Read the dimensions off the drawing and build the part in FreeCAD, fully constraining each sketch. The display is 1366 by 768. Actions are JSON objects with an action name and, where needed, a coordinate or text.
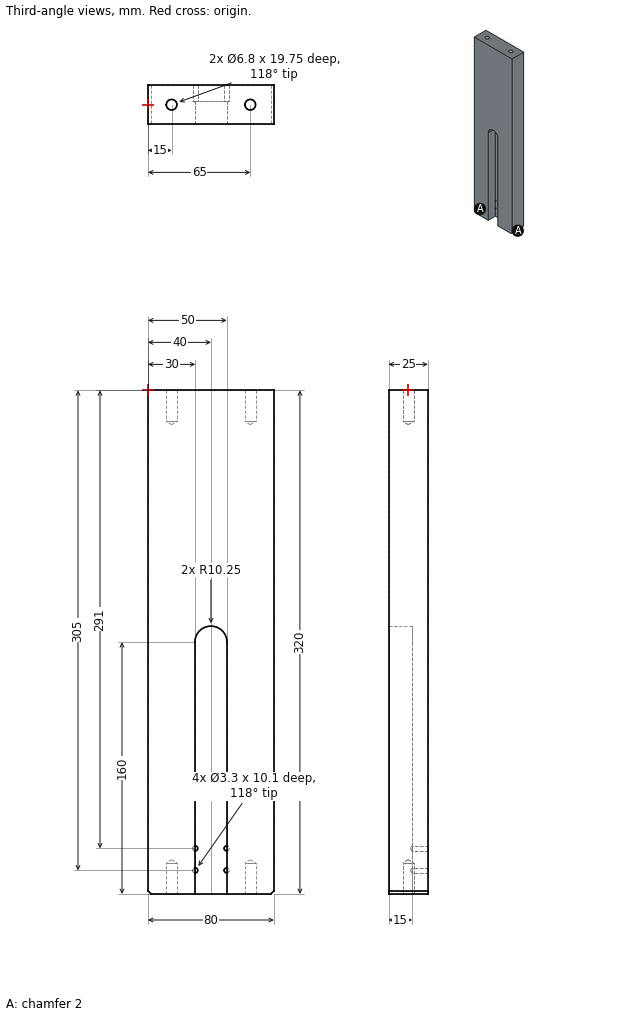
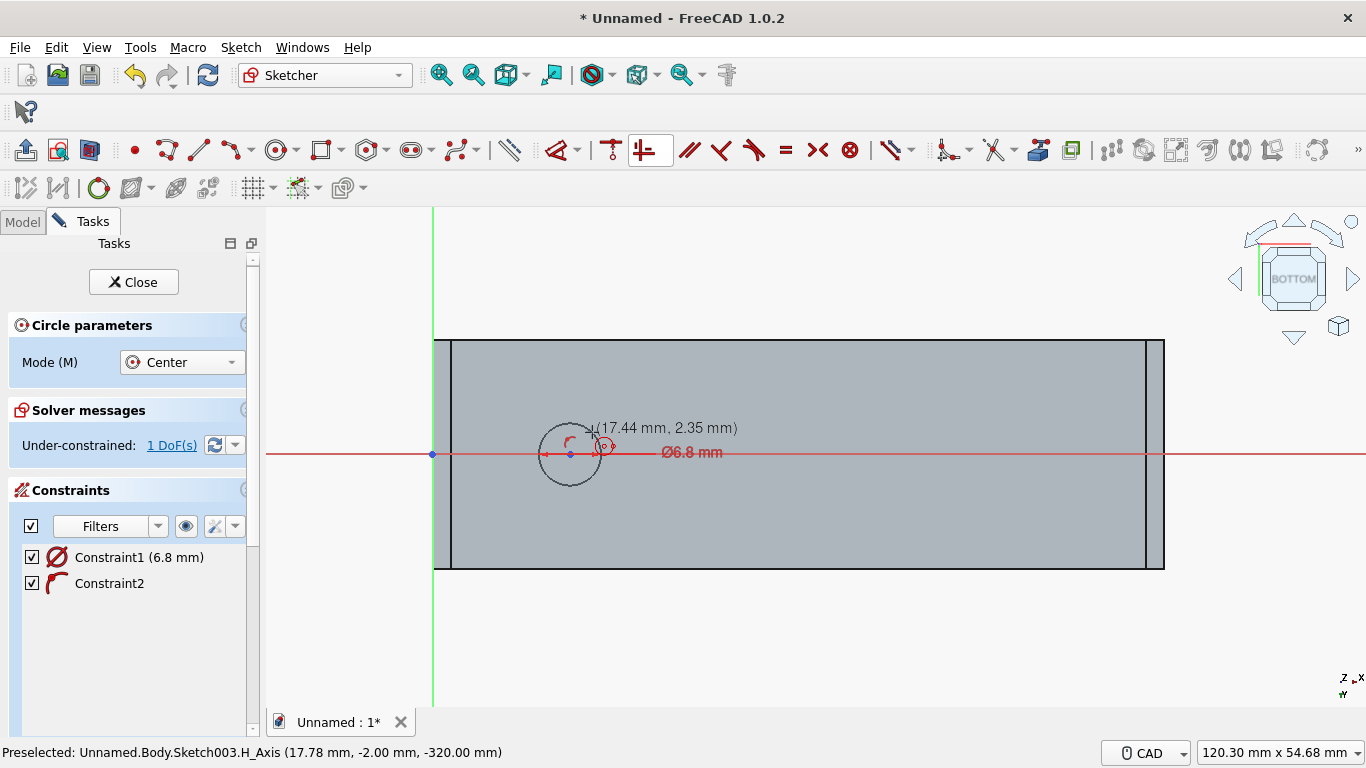
{"action": "left_click", "coordinate": [1027, 454]}
{"action": "mouse_move", "coordinate": [1049, 432]}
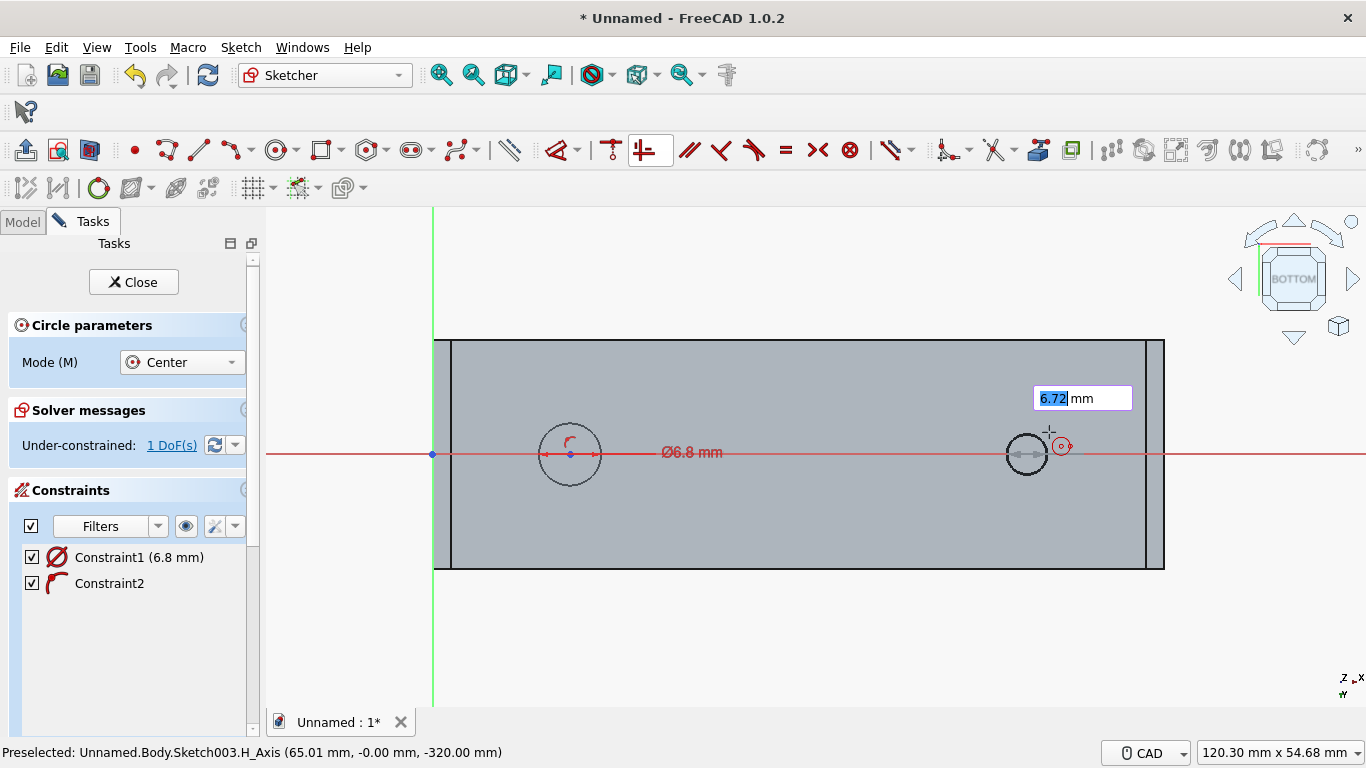
{"action": "type", "text": "6.8"}
{"action": "key", "text": "Return"}
{"action": "key", "text": "Escape"}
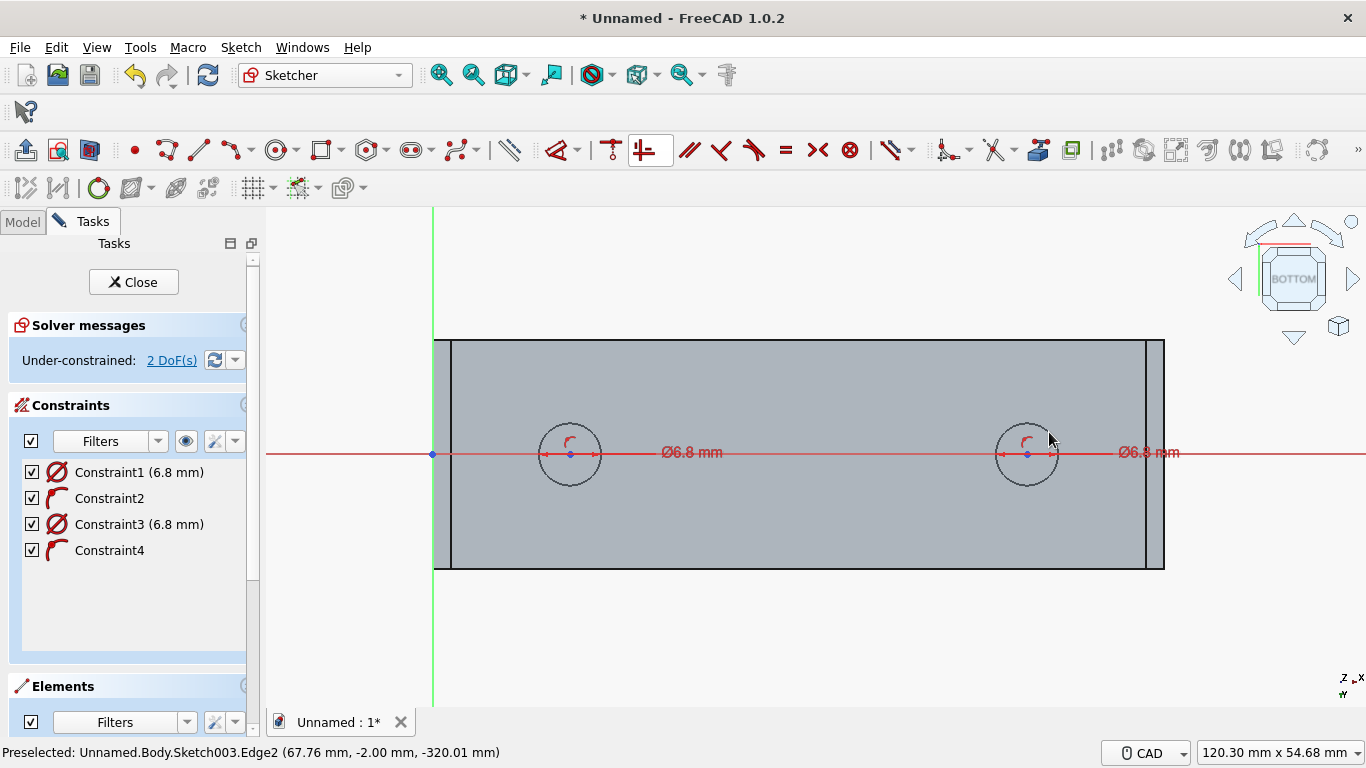
{"action": "key", "text": "d"}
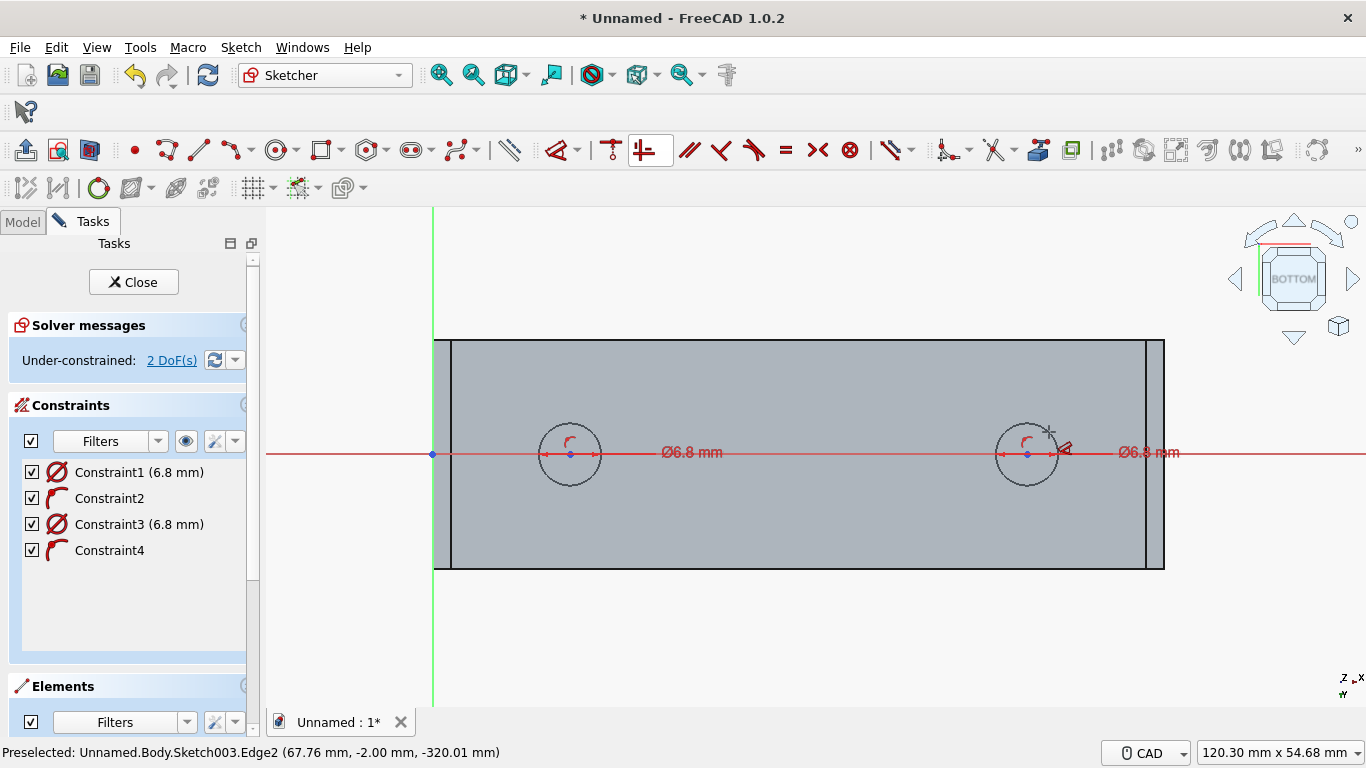
{"action": "left_click", "coordinate": [570, 454]}
{"action": "left_click", "coordinate": [501, 488]}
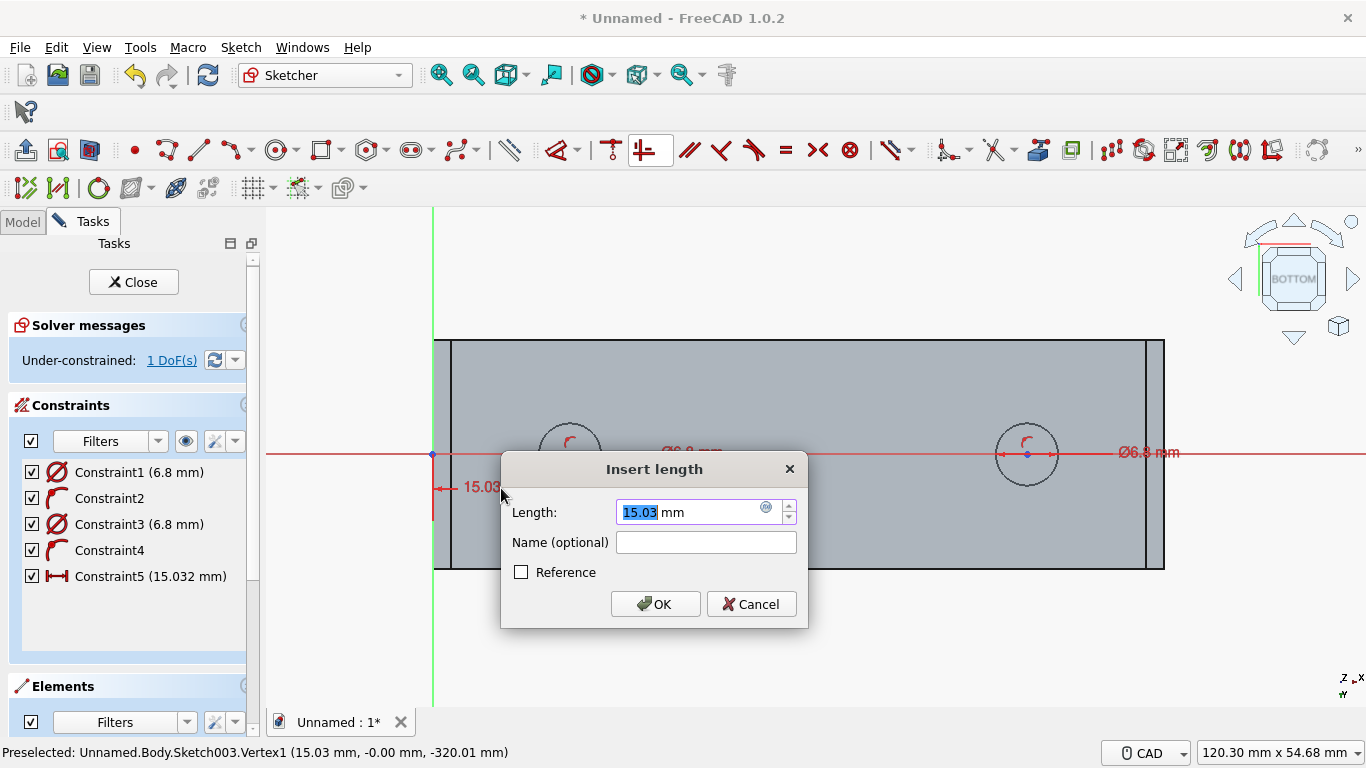
{"action": "type", "text": "15"}
{"action": "key", "text": "Return"}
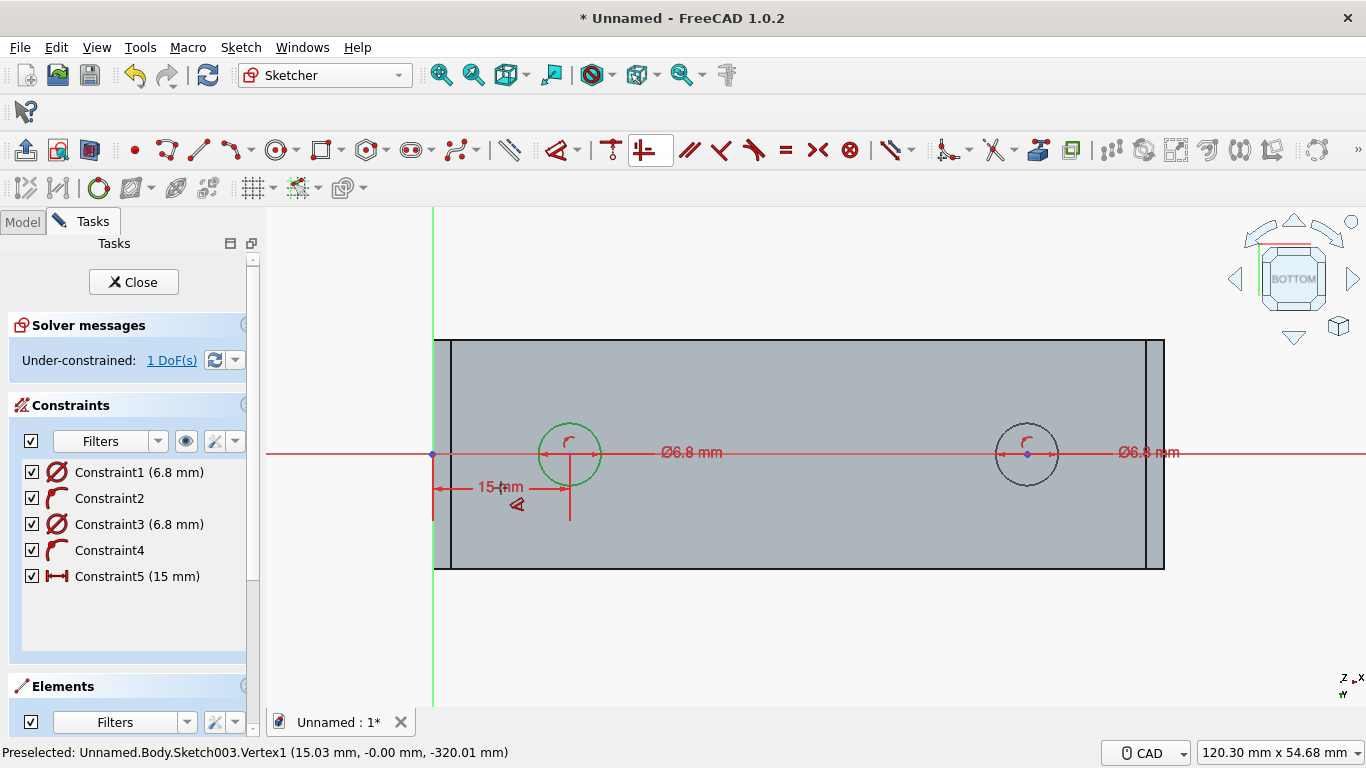
{"action": "left_click", "coordinate": [1027, 454]}
{"action": "left_click", "coordinate": [730, 488]}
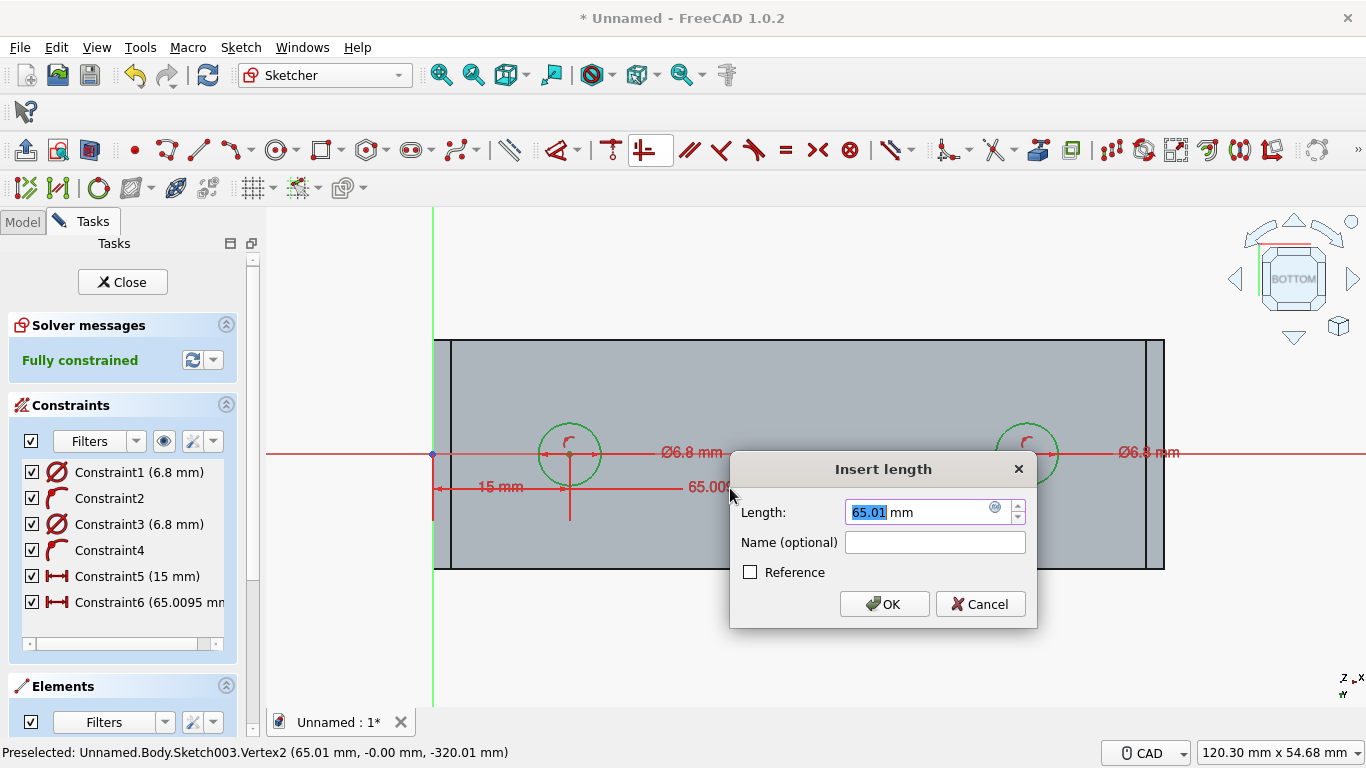
{"action": "type", "text": "65"}
{"action": "key", "text": "Return"}
{"action": "key", "text": "Escape"}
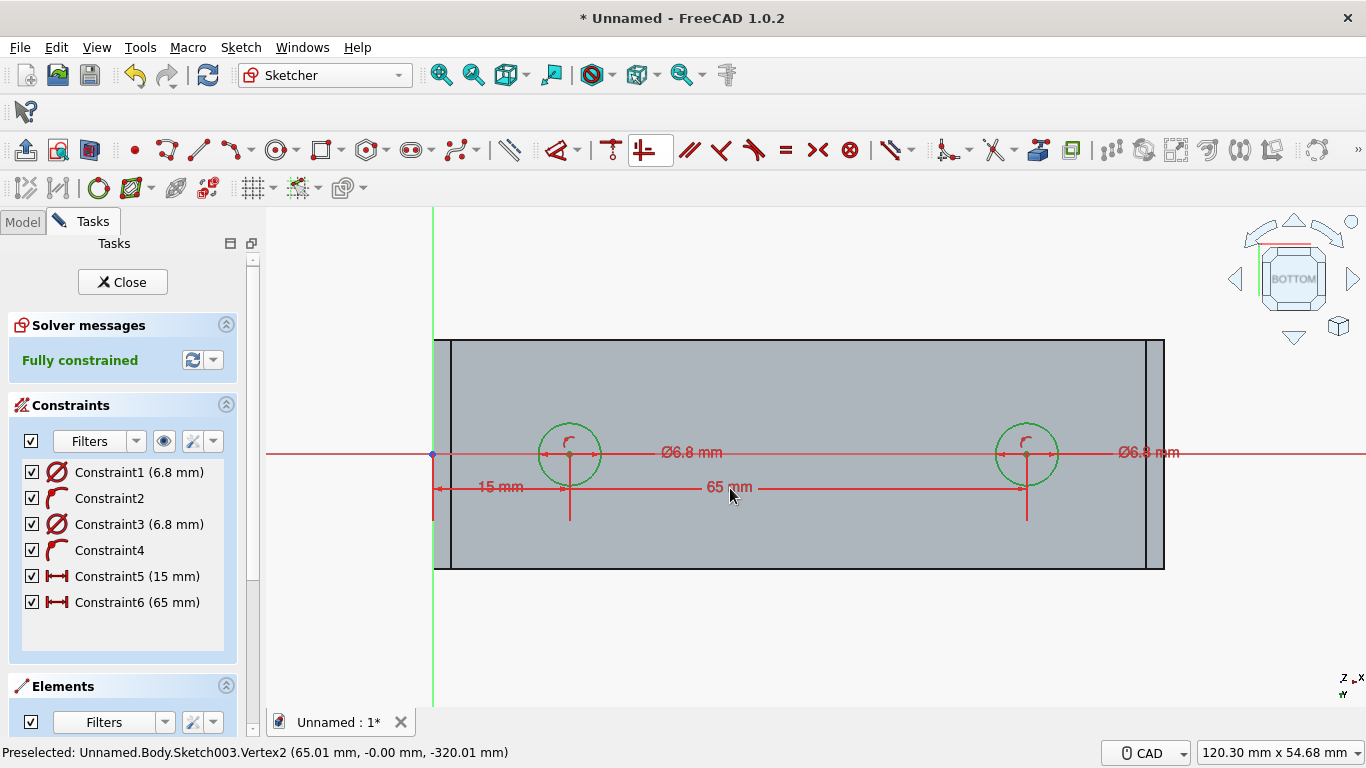
{"action": "left_click", "coordinate": [123, 282]}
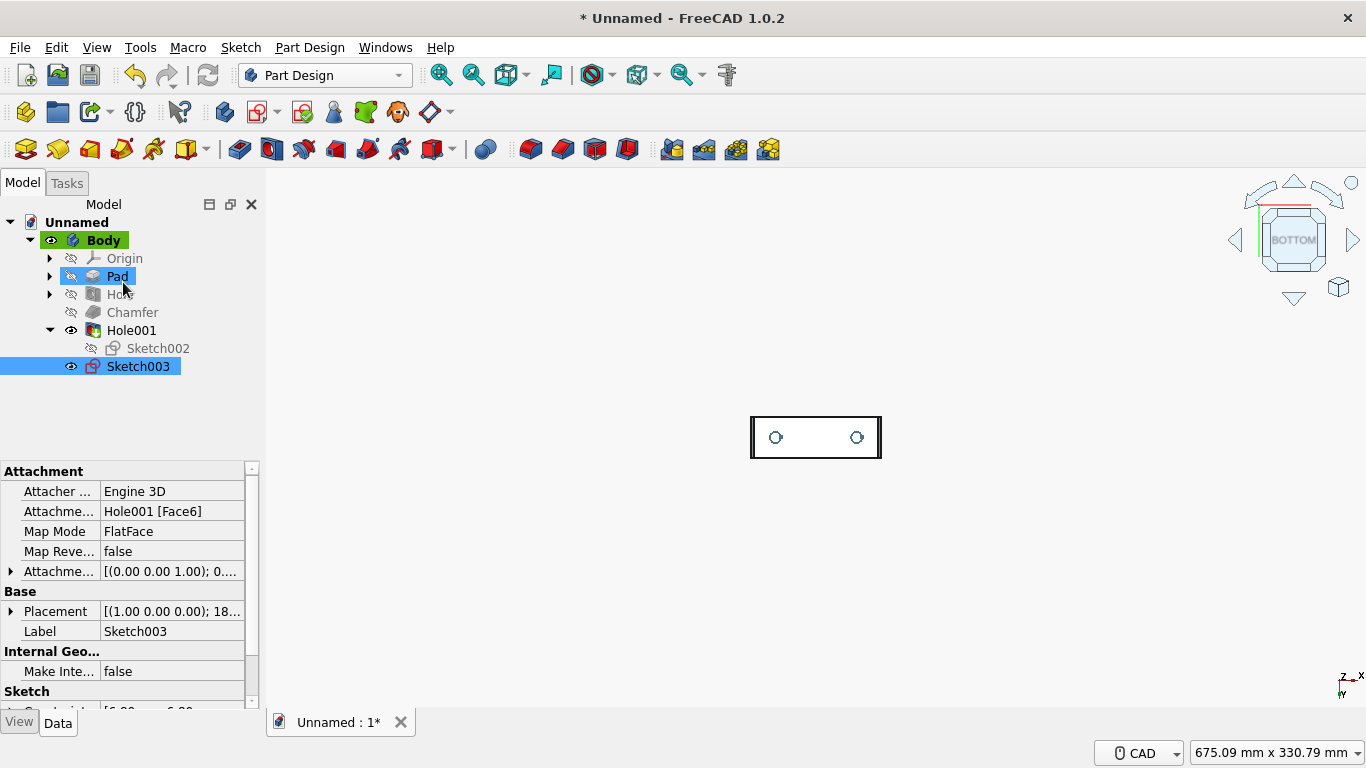
{"action": "left_click", "coordinate": [272, 150]}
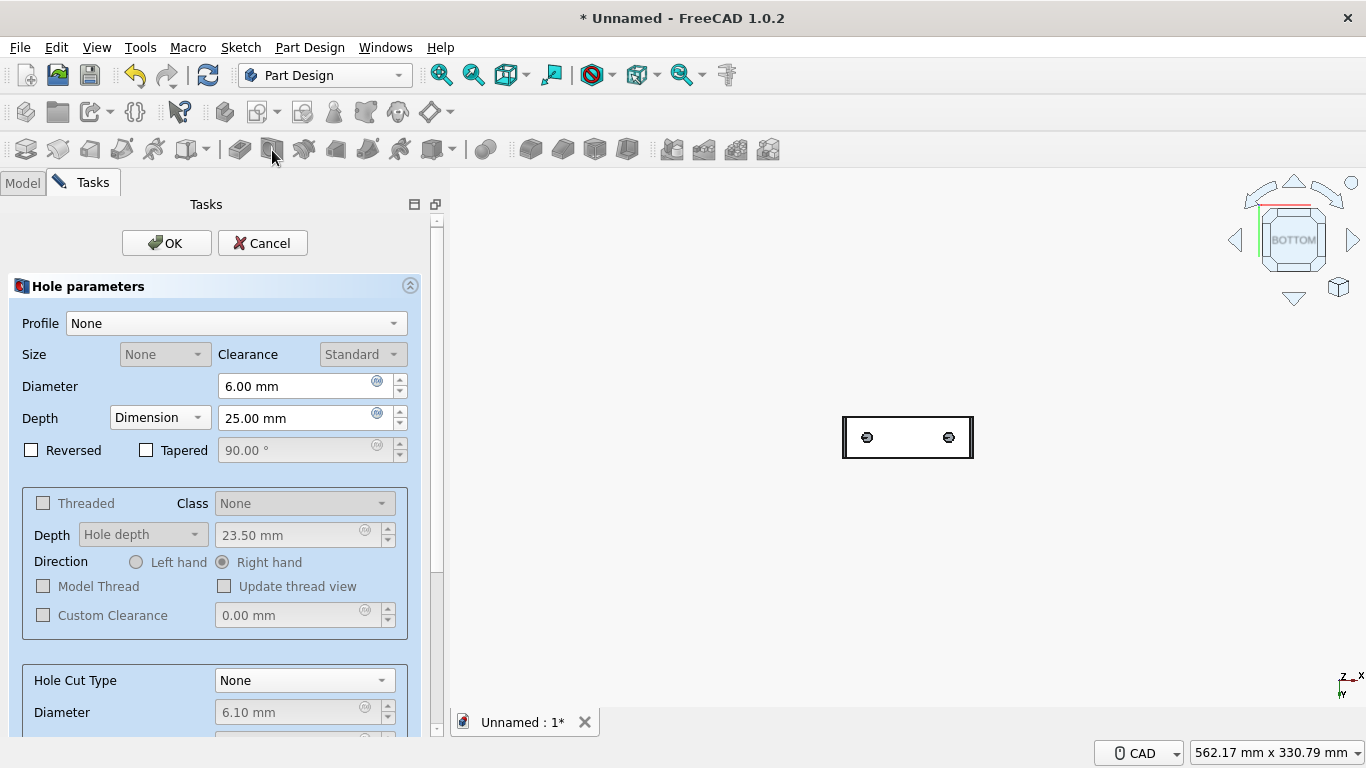
{"action": "triple_click", "coordinate": [305, 386]}